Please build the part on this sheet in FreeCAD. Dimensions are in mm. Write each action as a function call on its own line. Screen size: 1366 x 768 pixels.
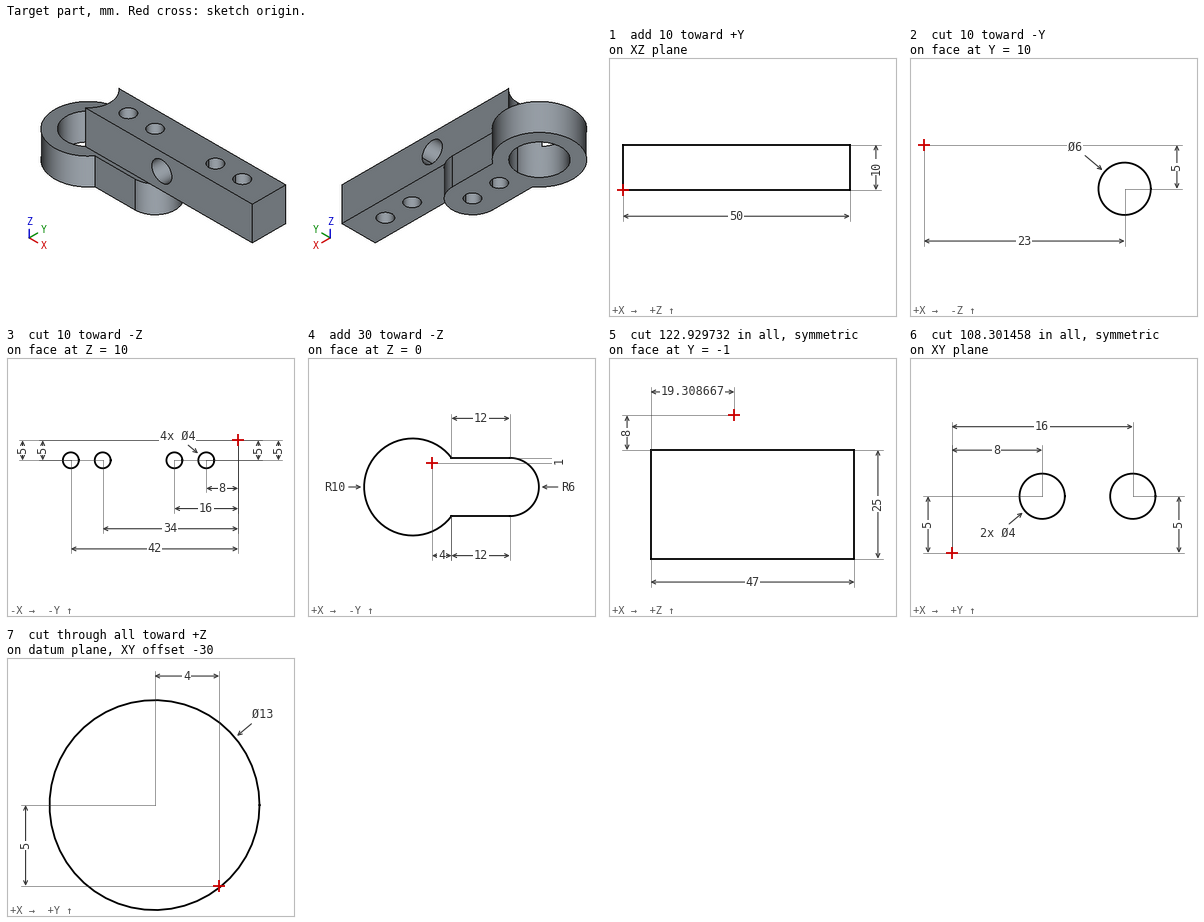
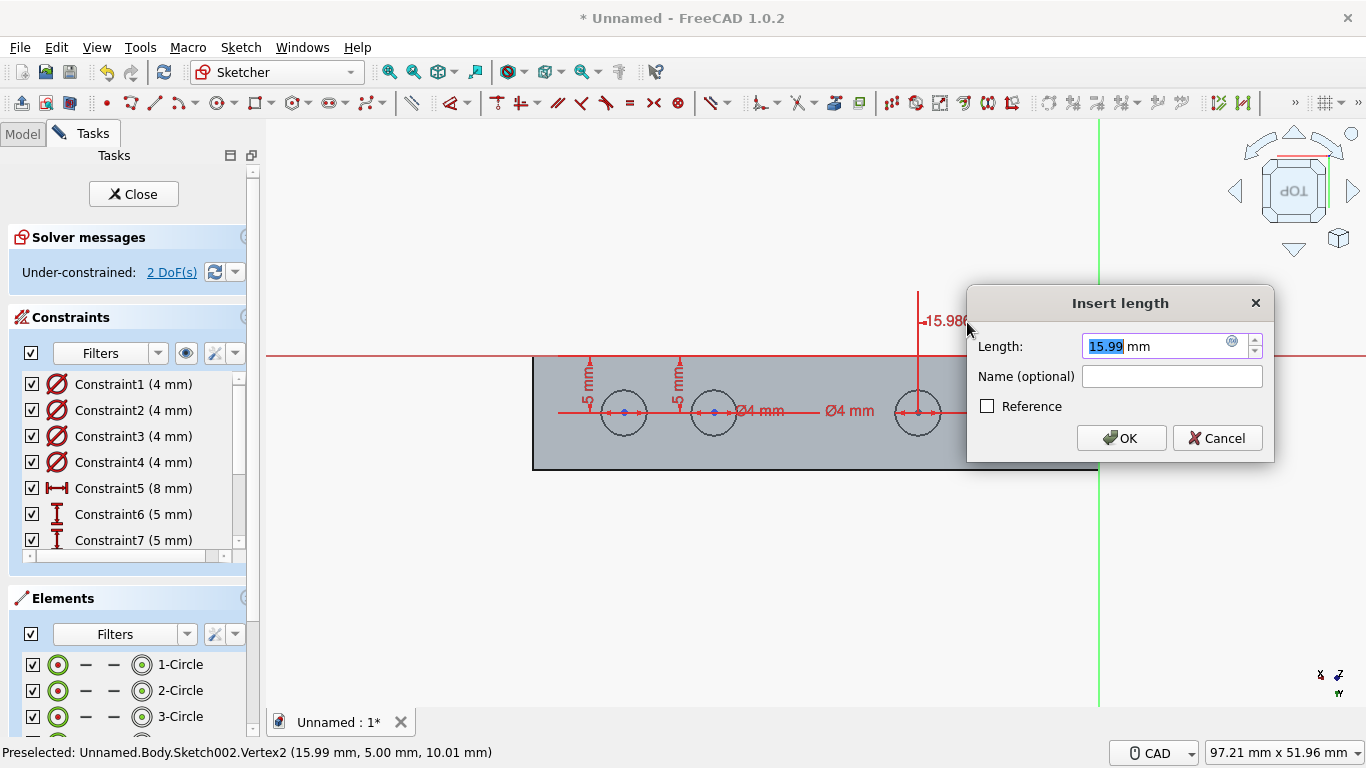
text(16)
key(Return)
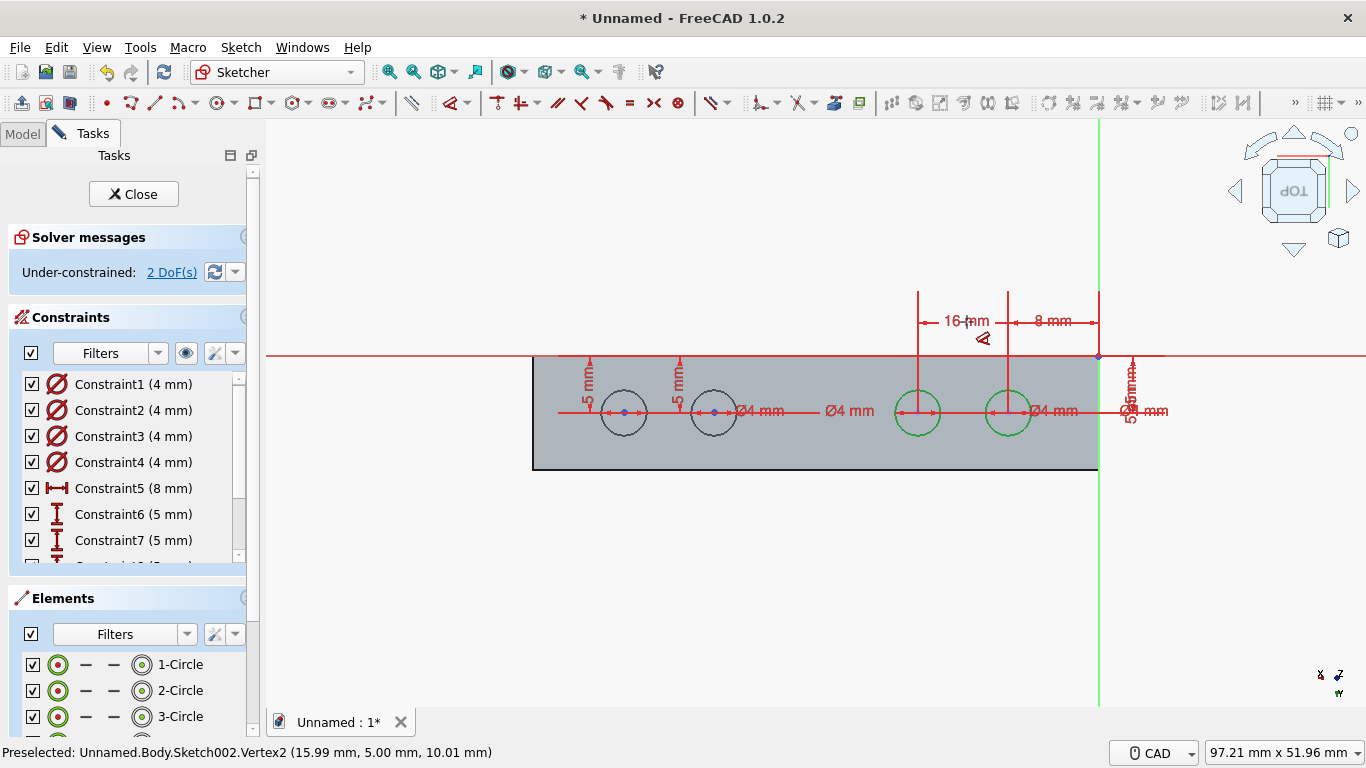
click(624, 413)
click(861, 322)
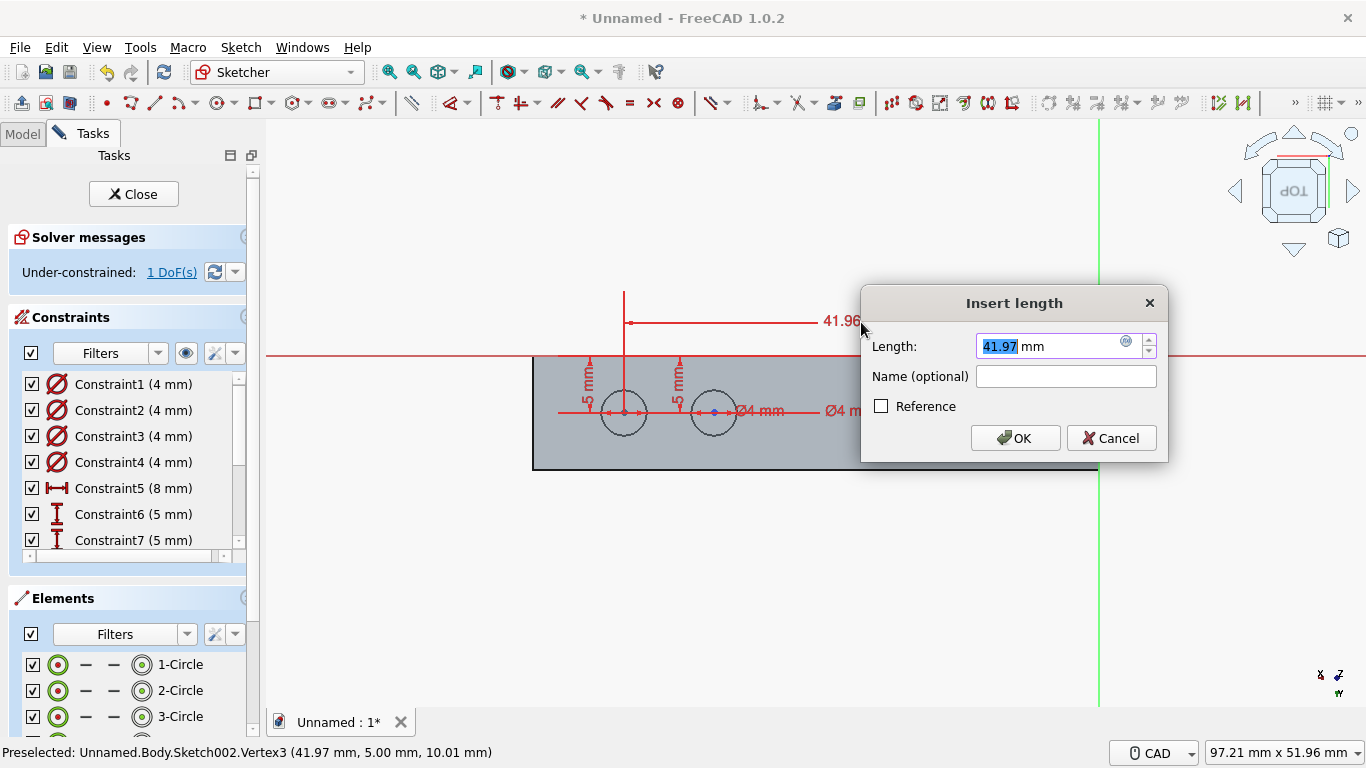
text(42)
key(Return)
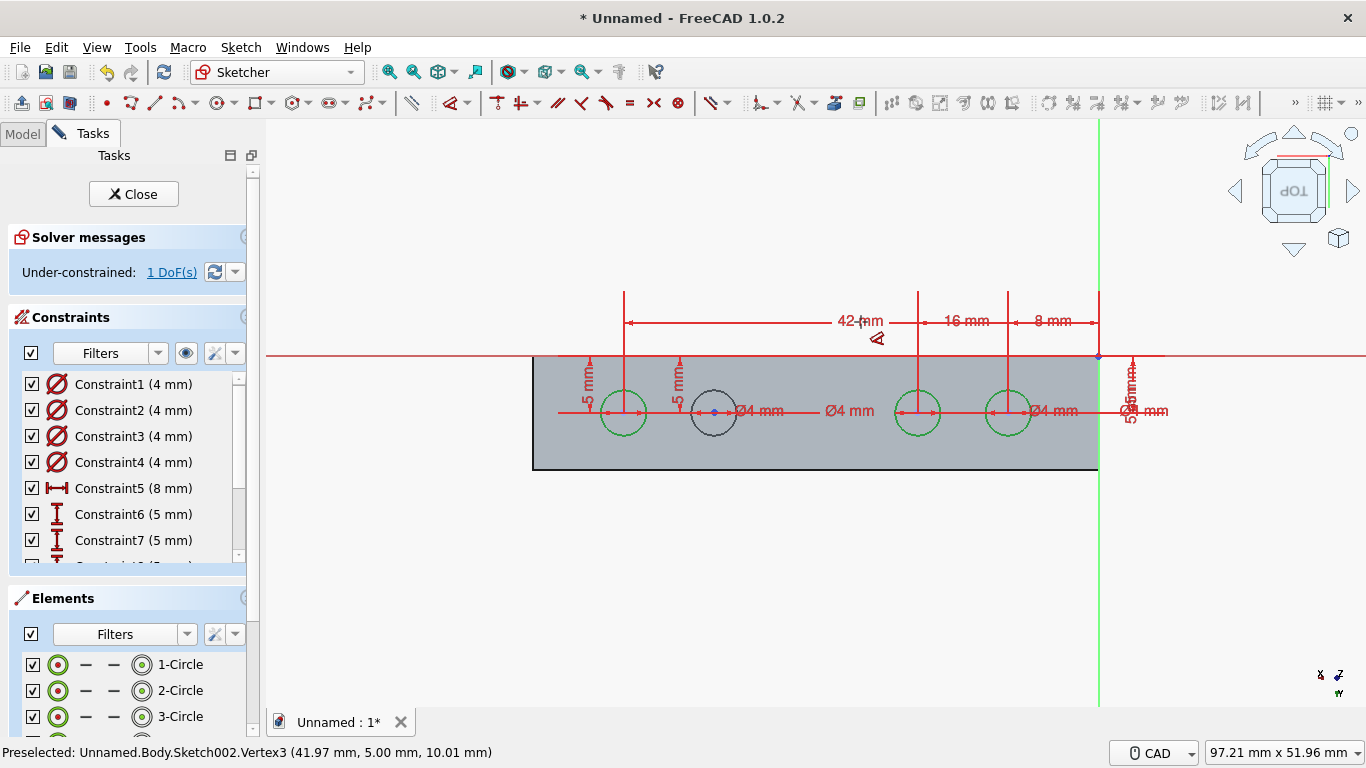
click(714, 413)
click(772, 322)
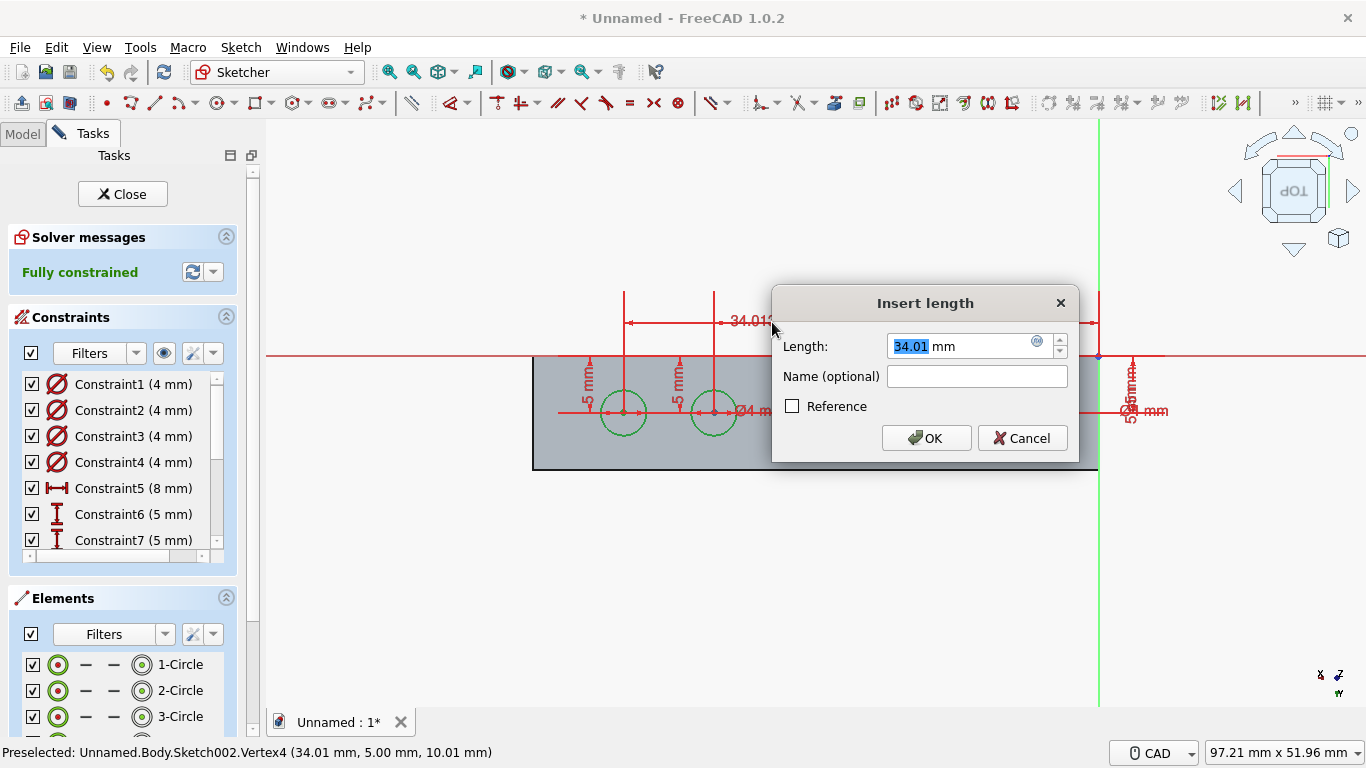
text(34)
key(Return)
key(Escape)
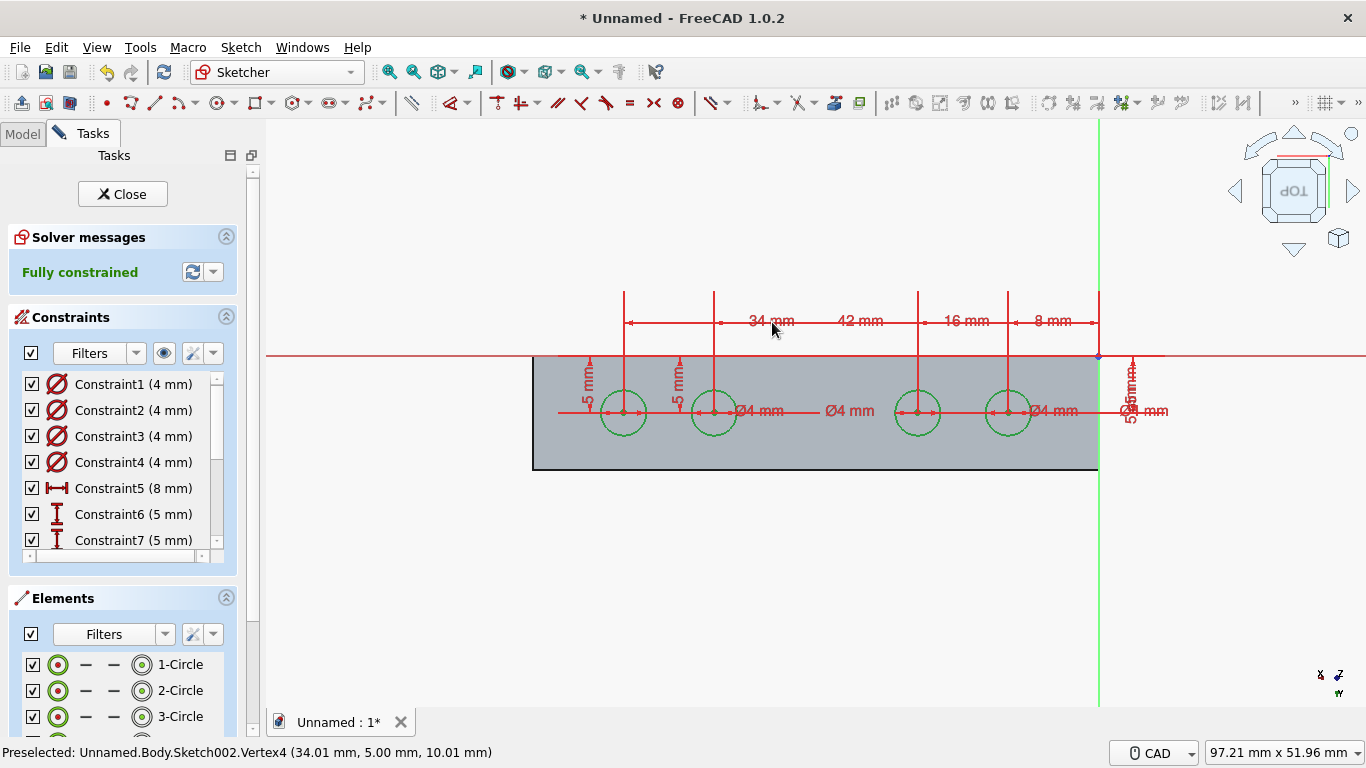
click(123, 194)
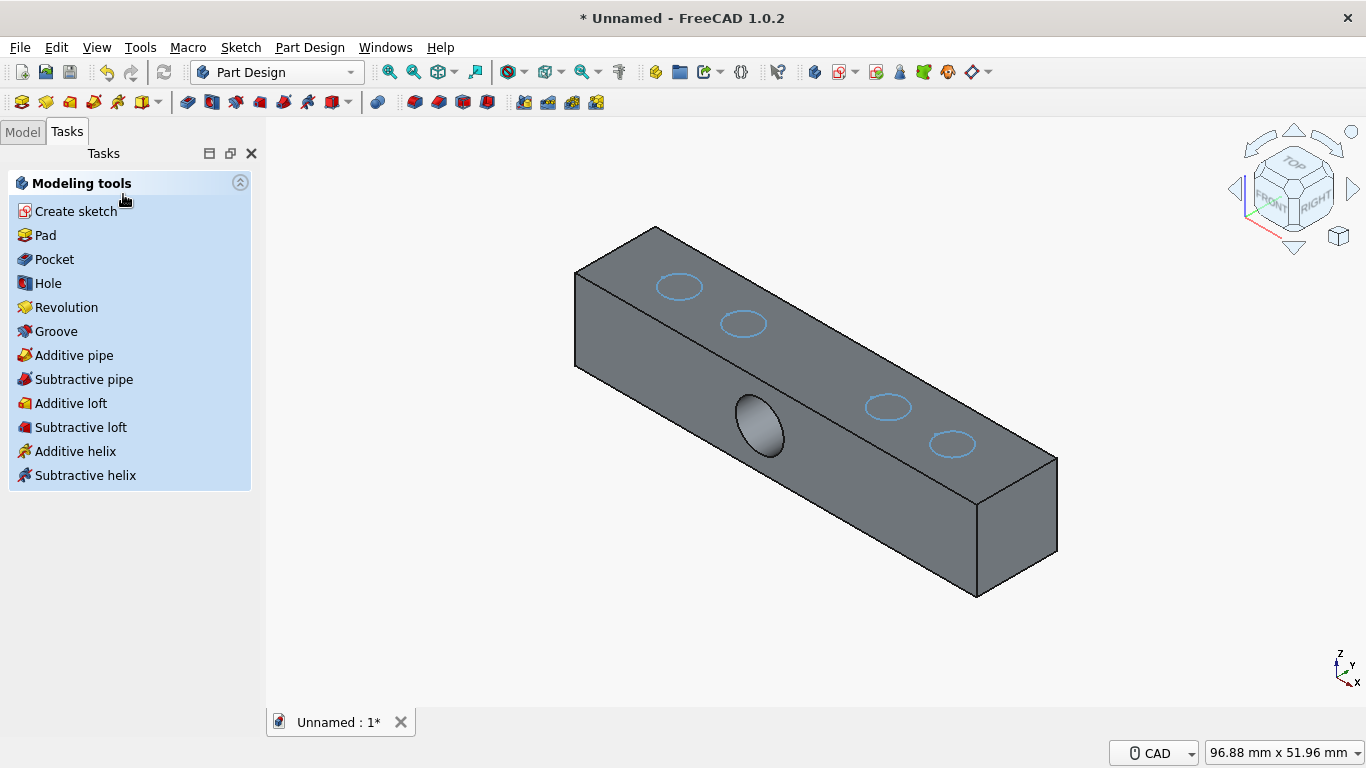
click(188, 102)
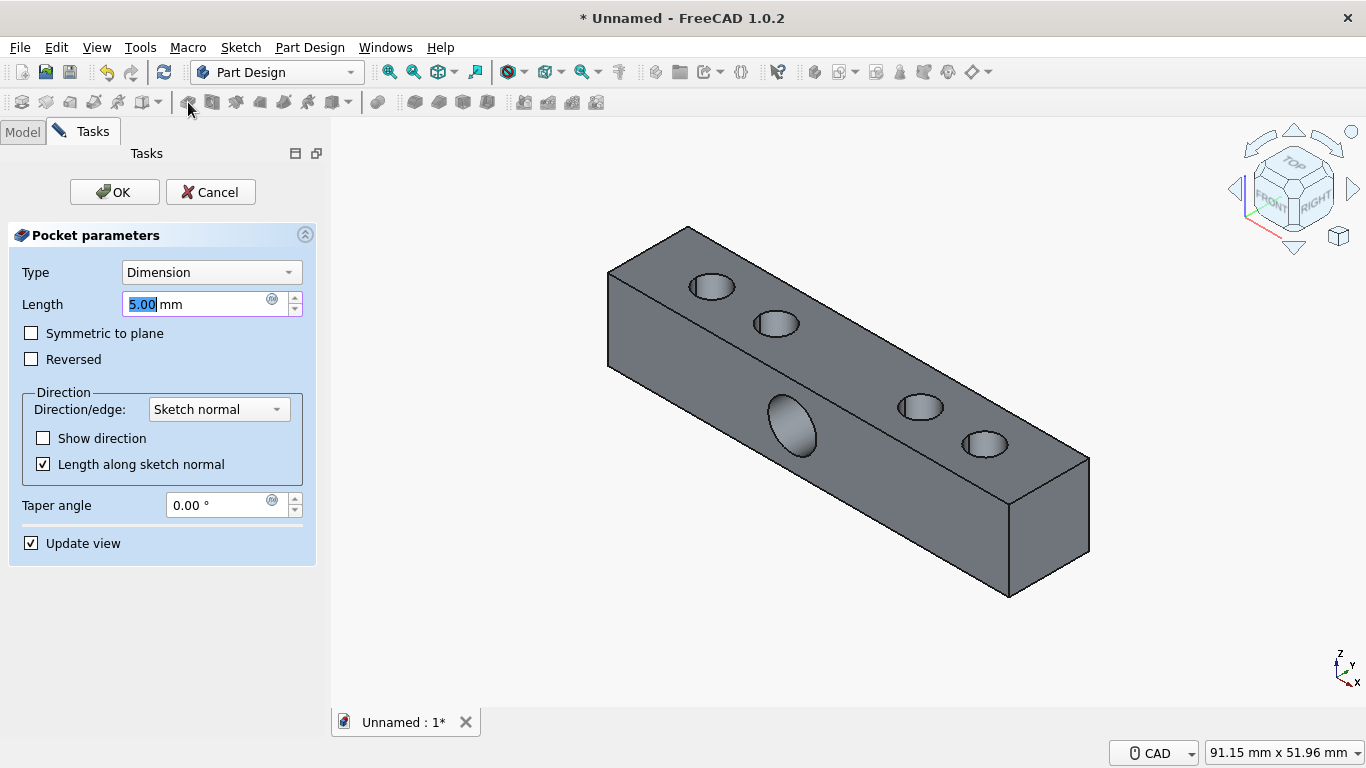
text(10)
key(Tab)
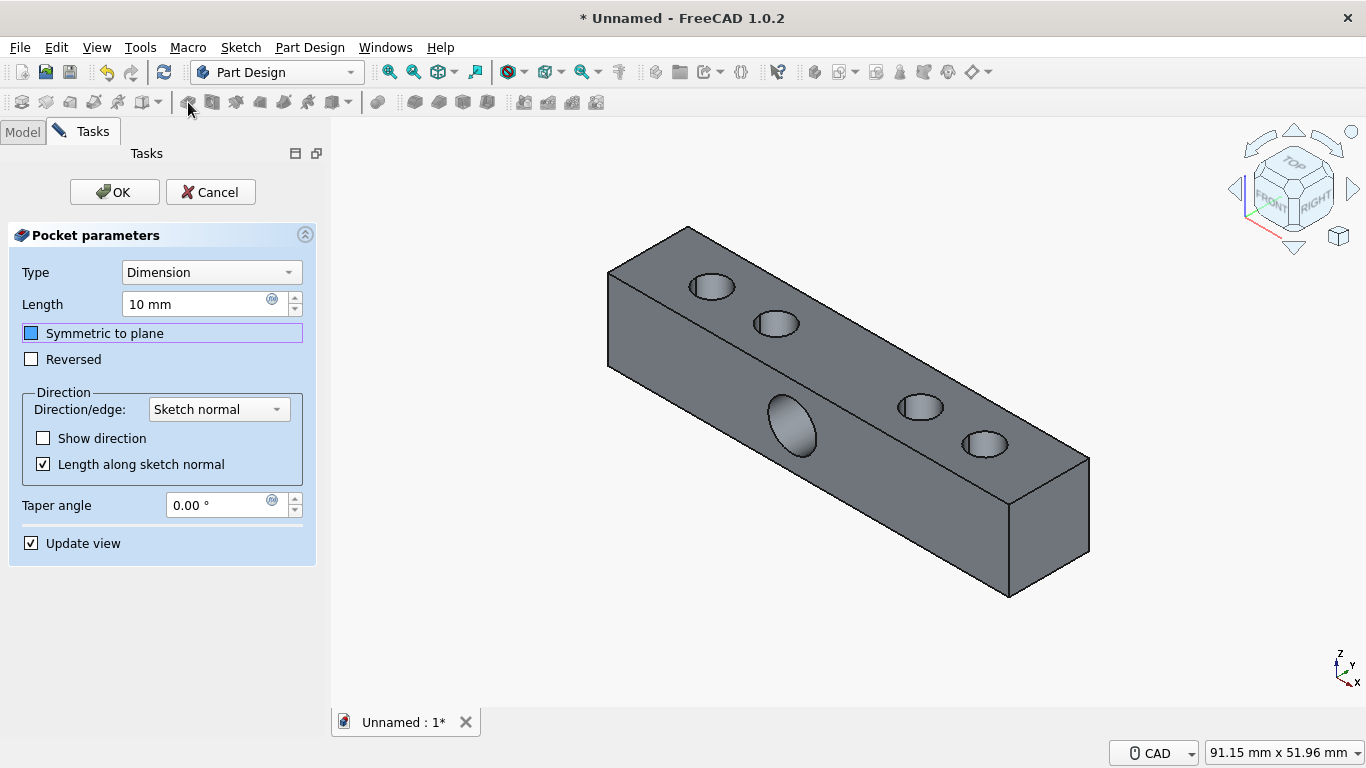
click(115, 192)